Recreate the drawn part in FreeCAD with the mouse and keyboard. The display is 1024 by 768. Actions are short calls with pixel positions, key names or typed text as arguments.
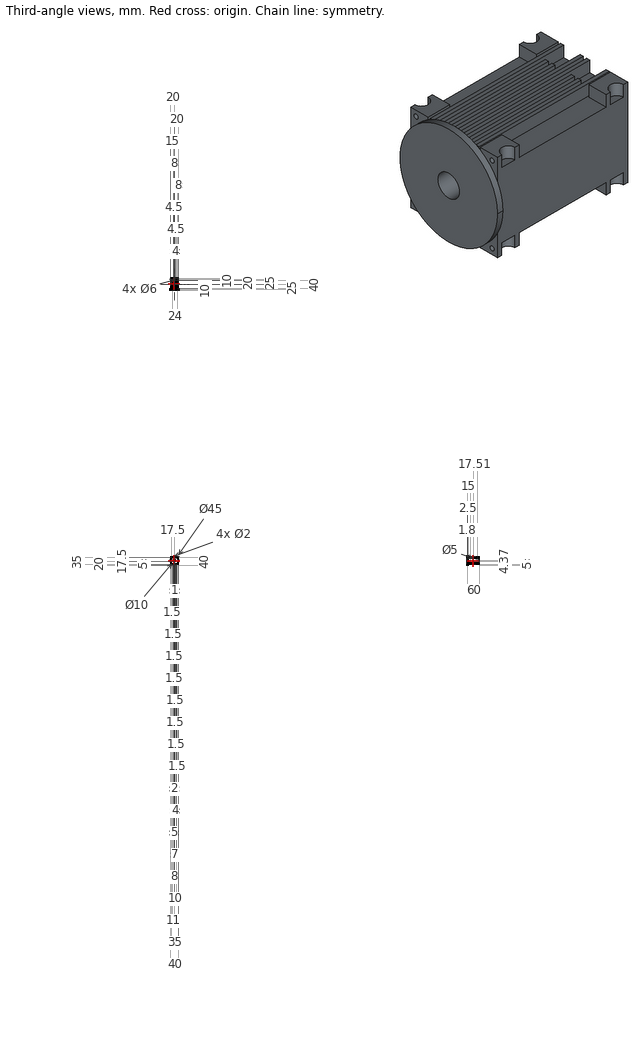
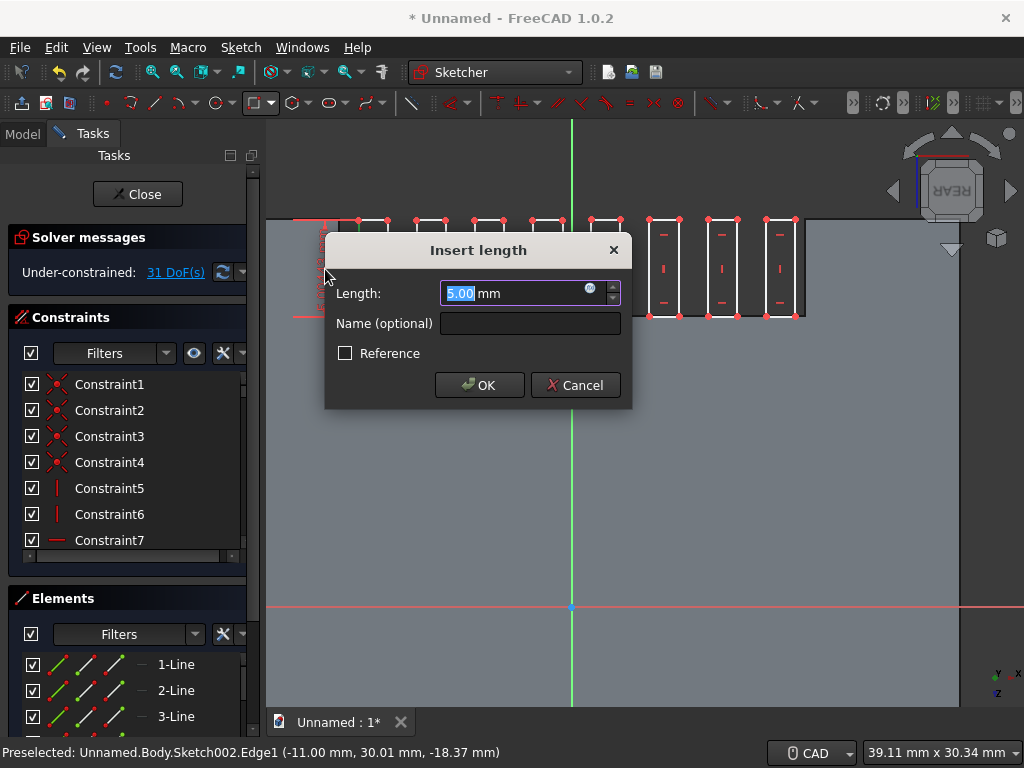
text(5)
key(Return)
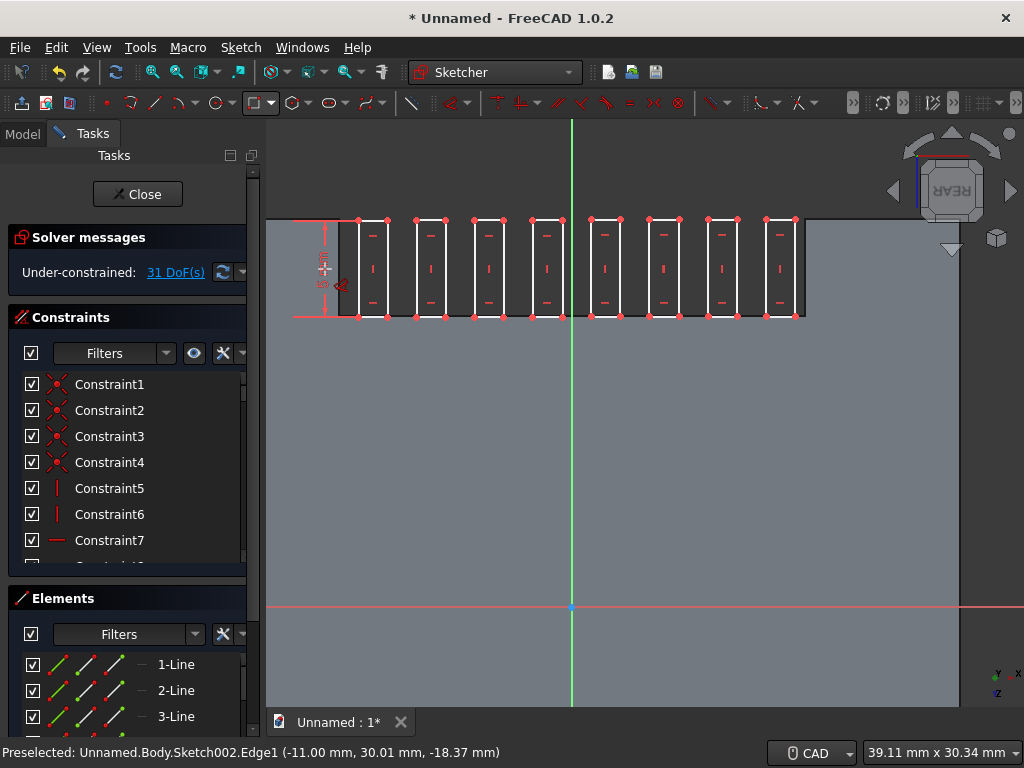
click(417, 250)
click(335, 247)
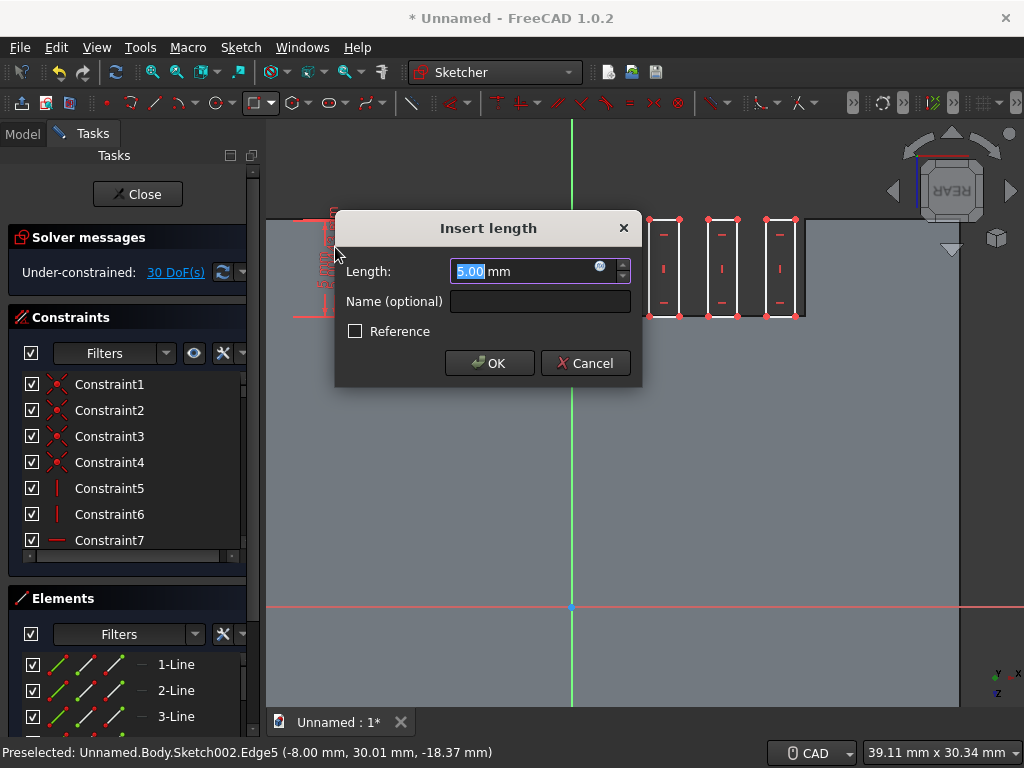
text(5)
key(Return)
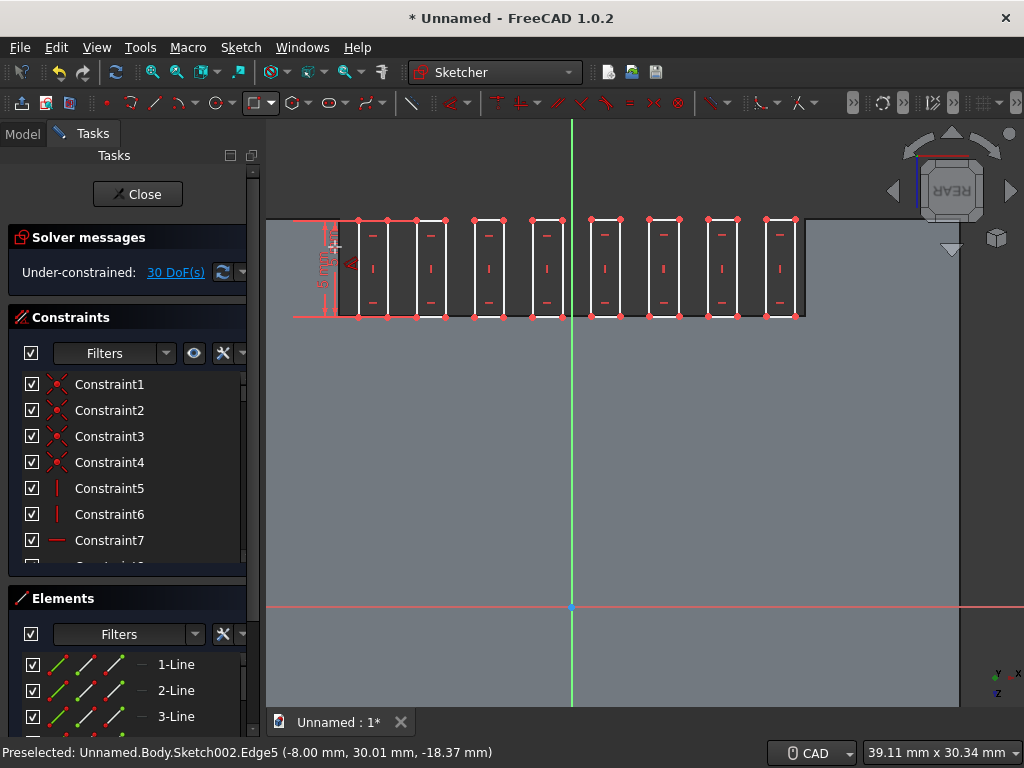
click(475, 250)
click(345, 291)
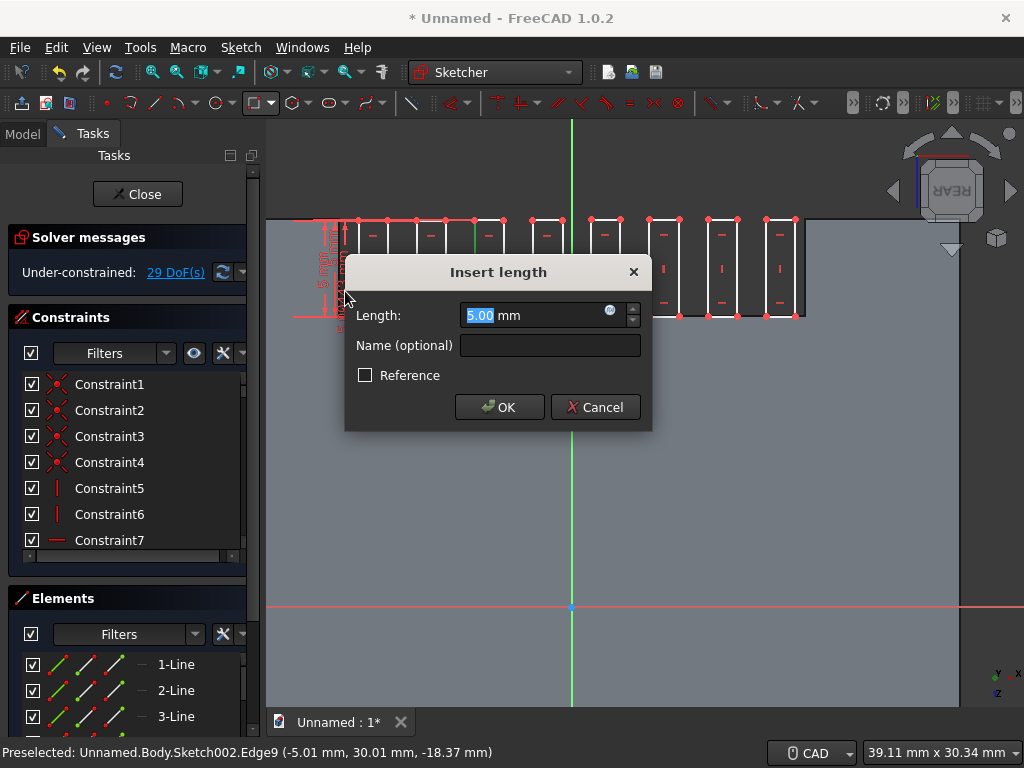
text(5)
key(Return)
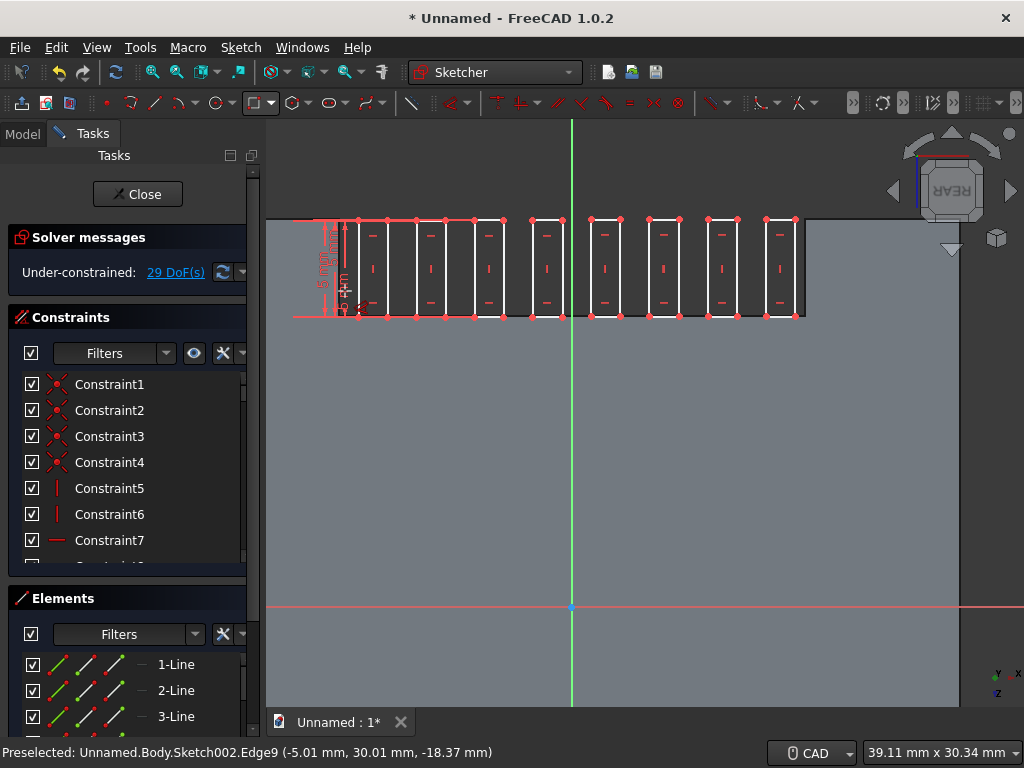
click(533, 249)
click(403, 269)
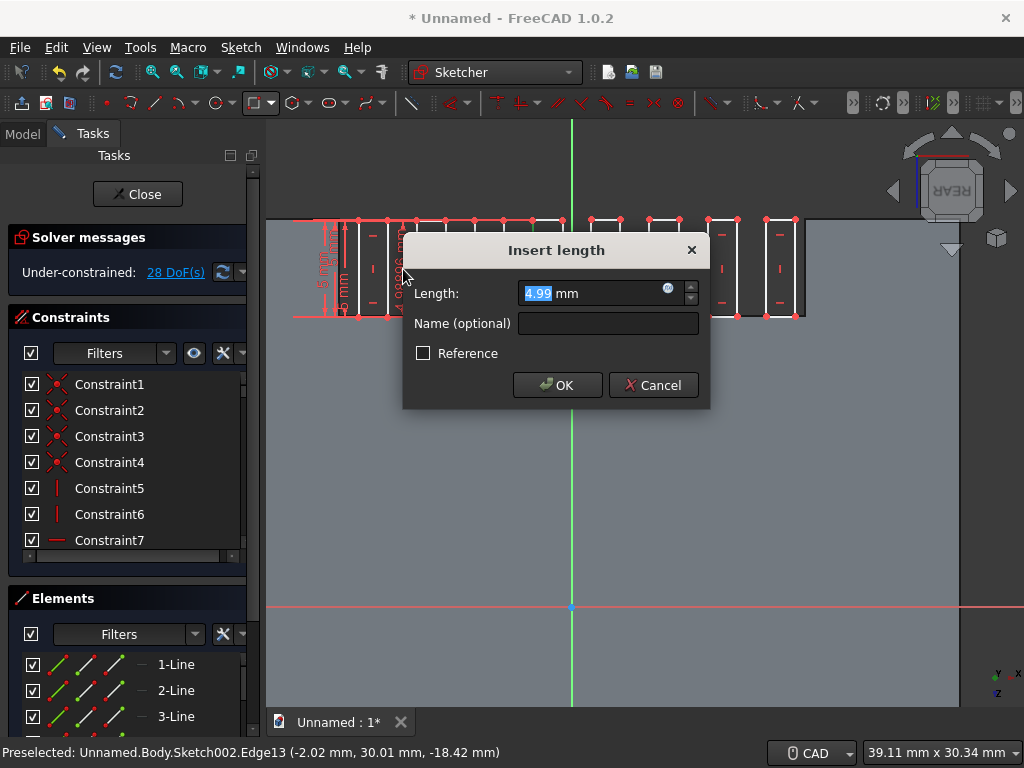
text(5)
key(Return)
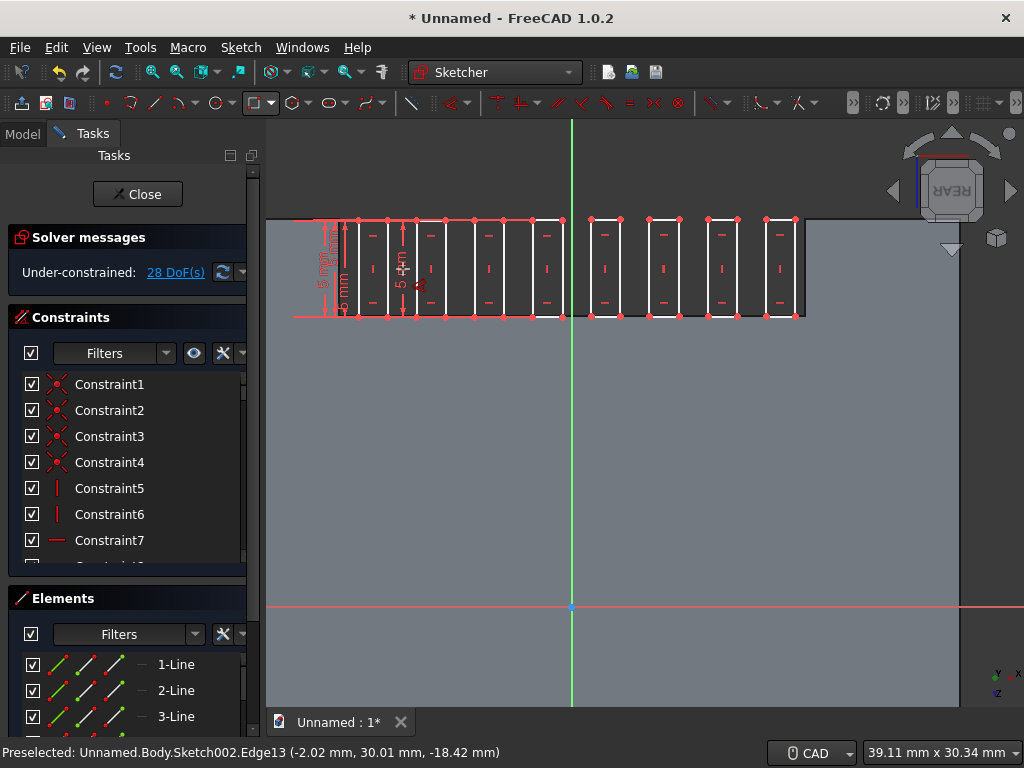
click(591, 249)
click(721, 269)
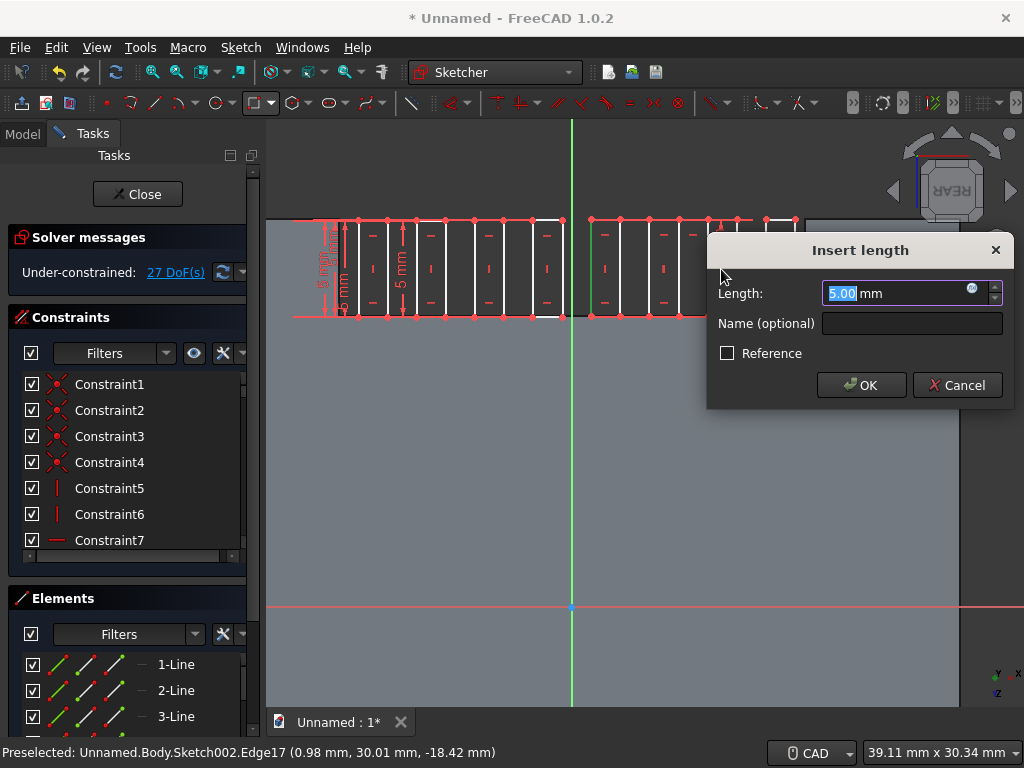
text(5)
key(Return)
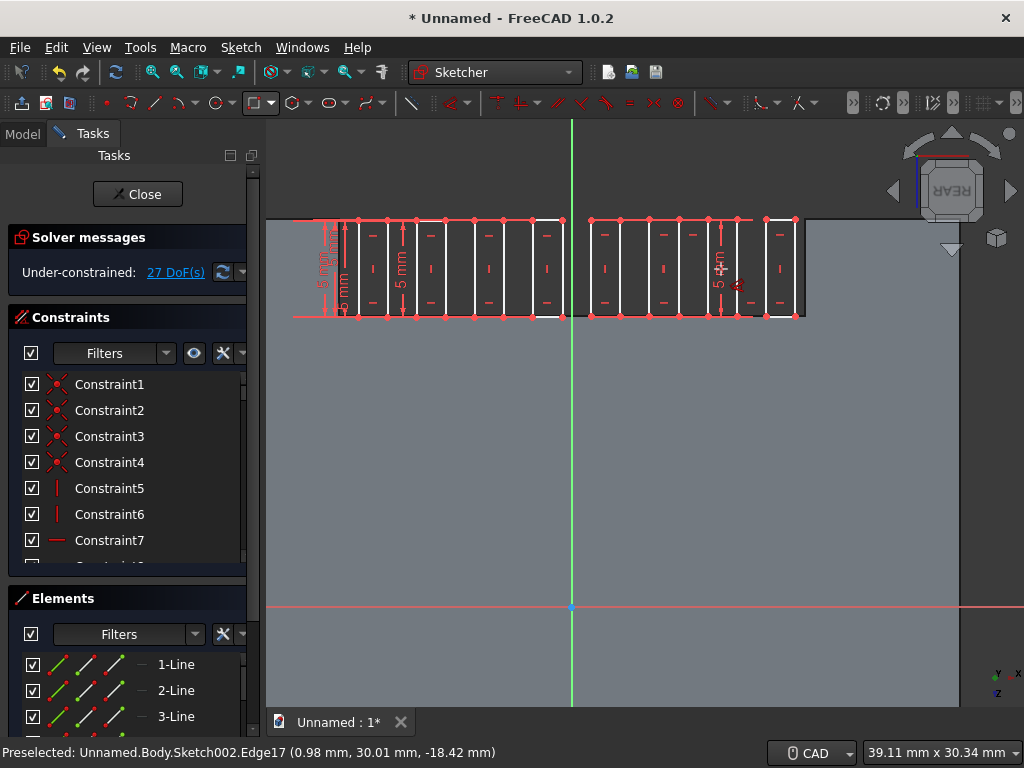
click(649, 249)
click(779, 246)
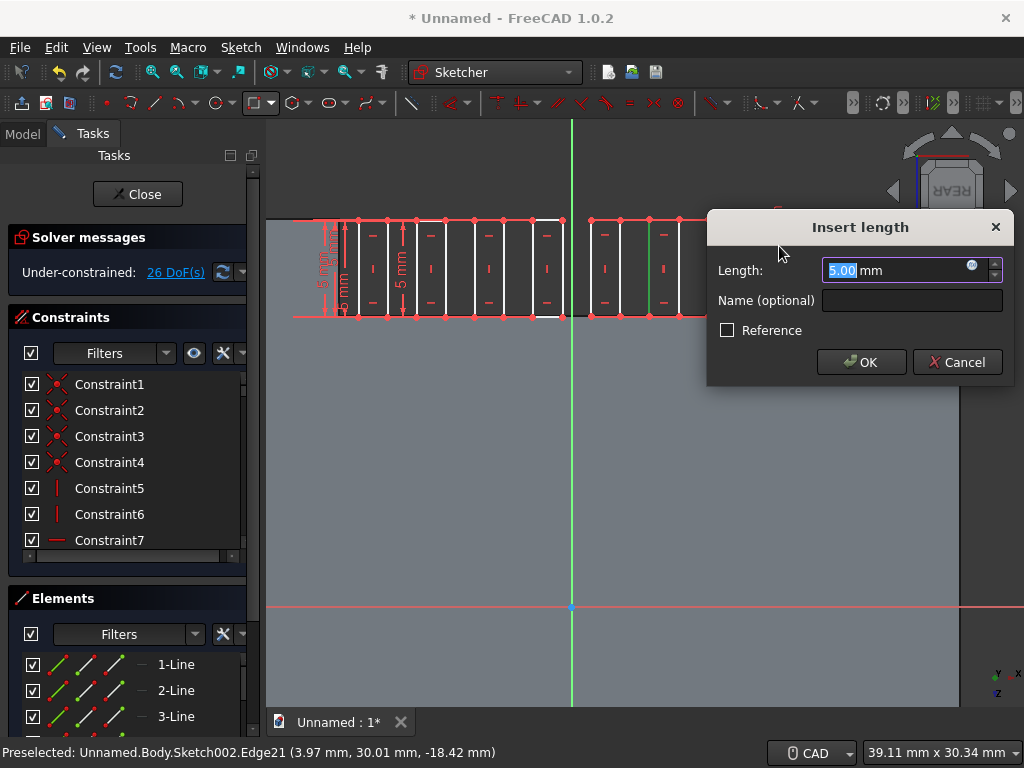
text(5)
key(Return)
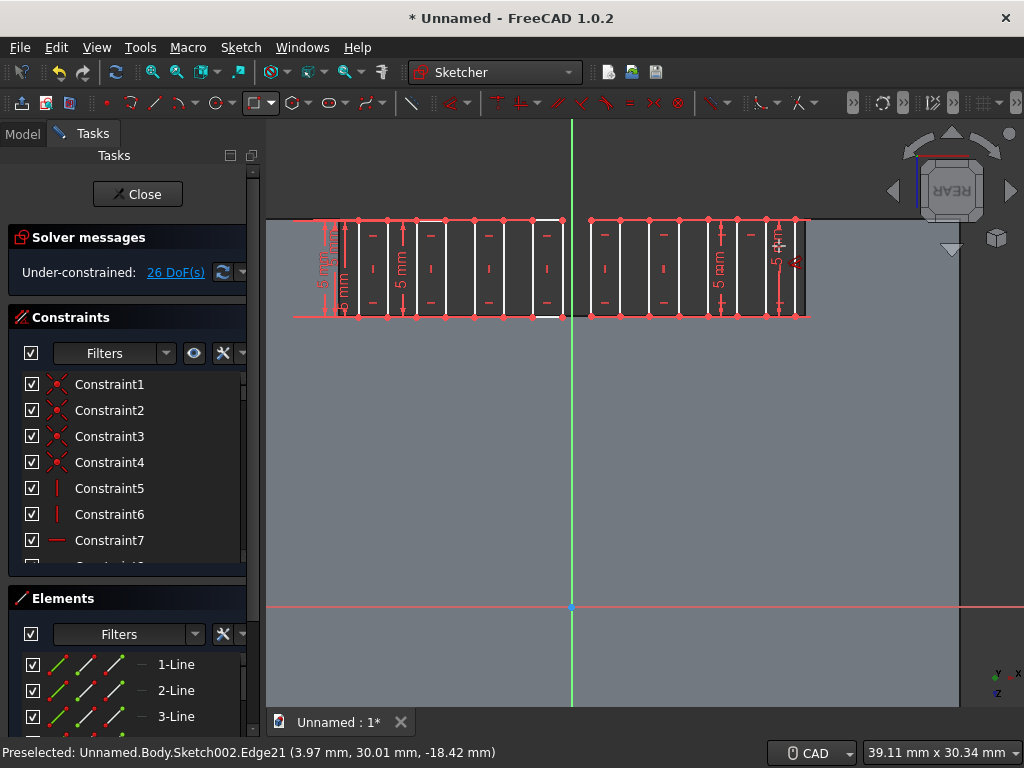
click(708, 249)
click(814, 269)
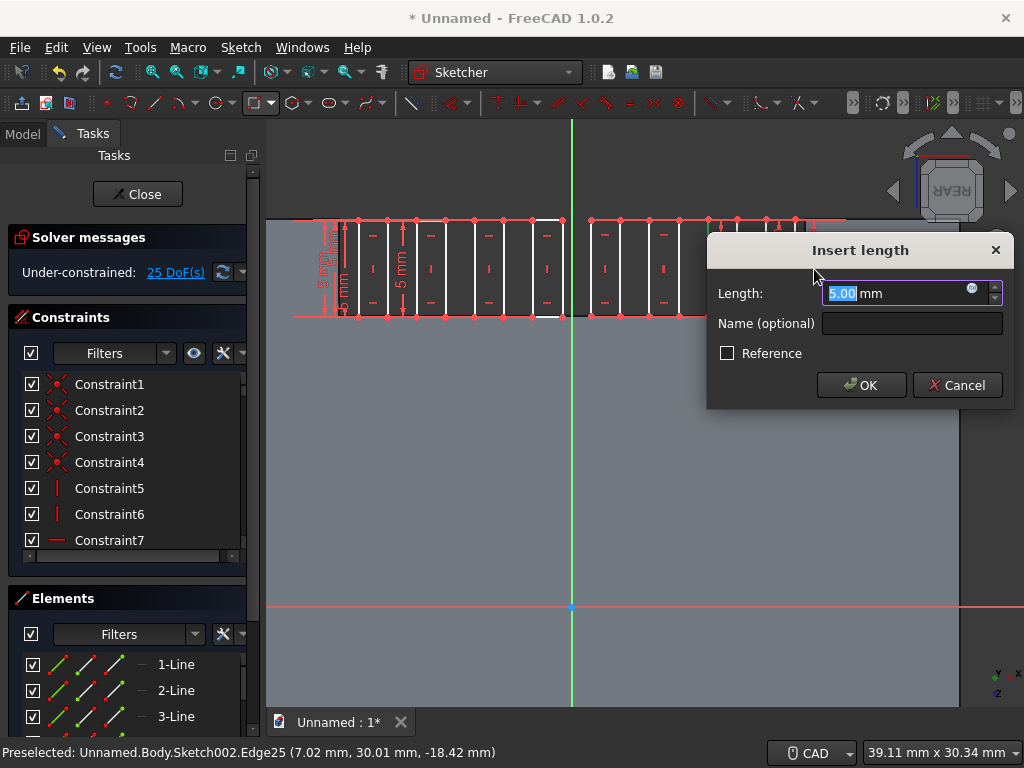
text(5)
key(Return)